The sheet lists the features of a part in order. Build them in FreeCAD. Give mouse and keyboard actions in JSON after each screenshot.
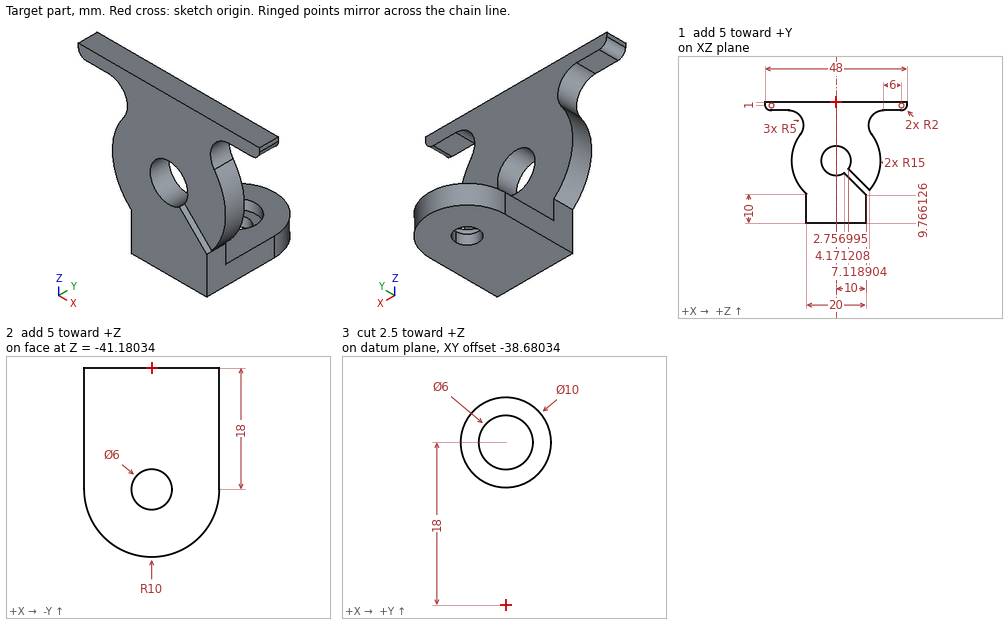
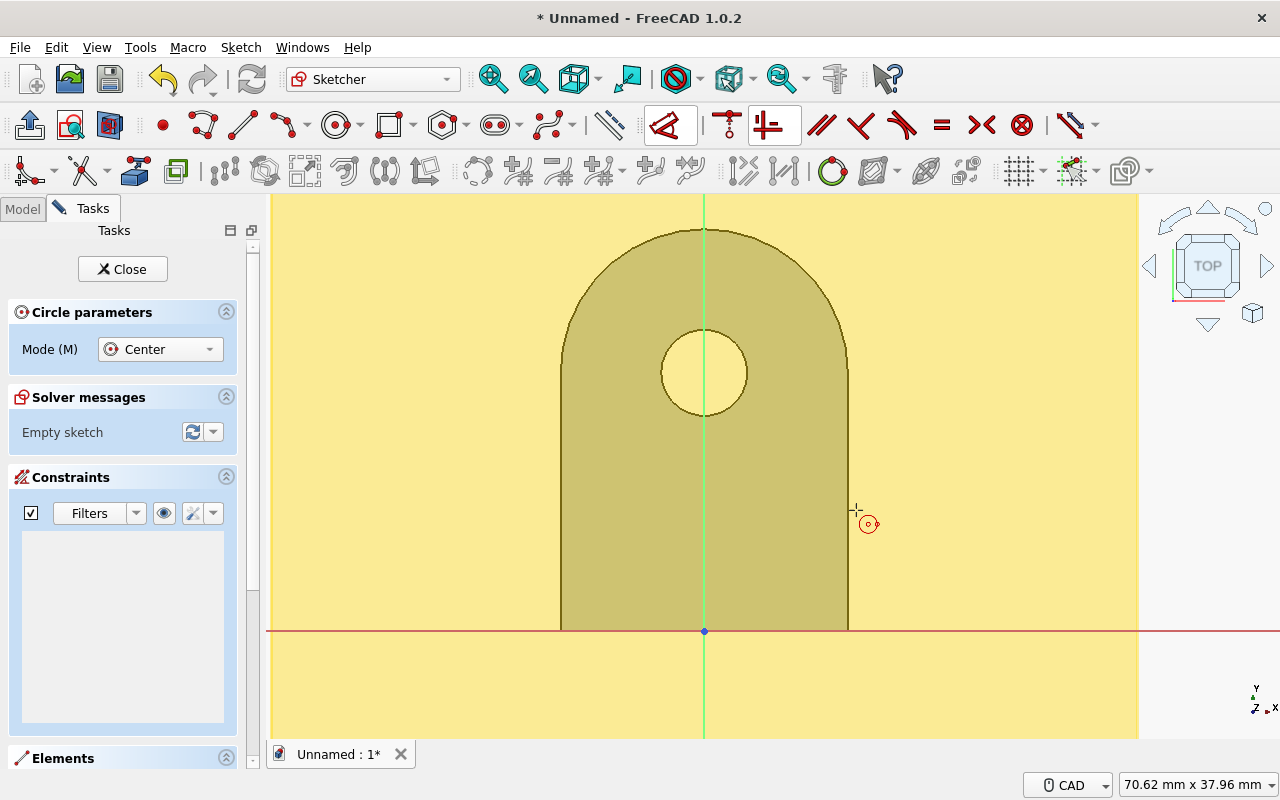
{"action": "left_click", "coordinate": [704, 373]}
{"action": "left_click", "coordinate": [755, 322]}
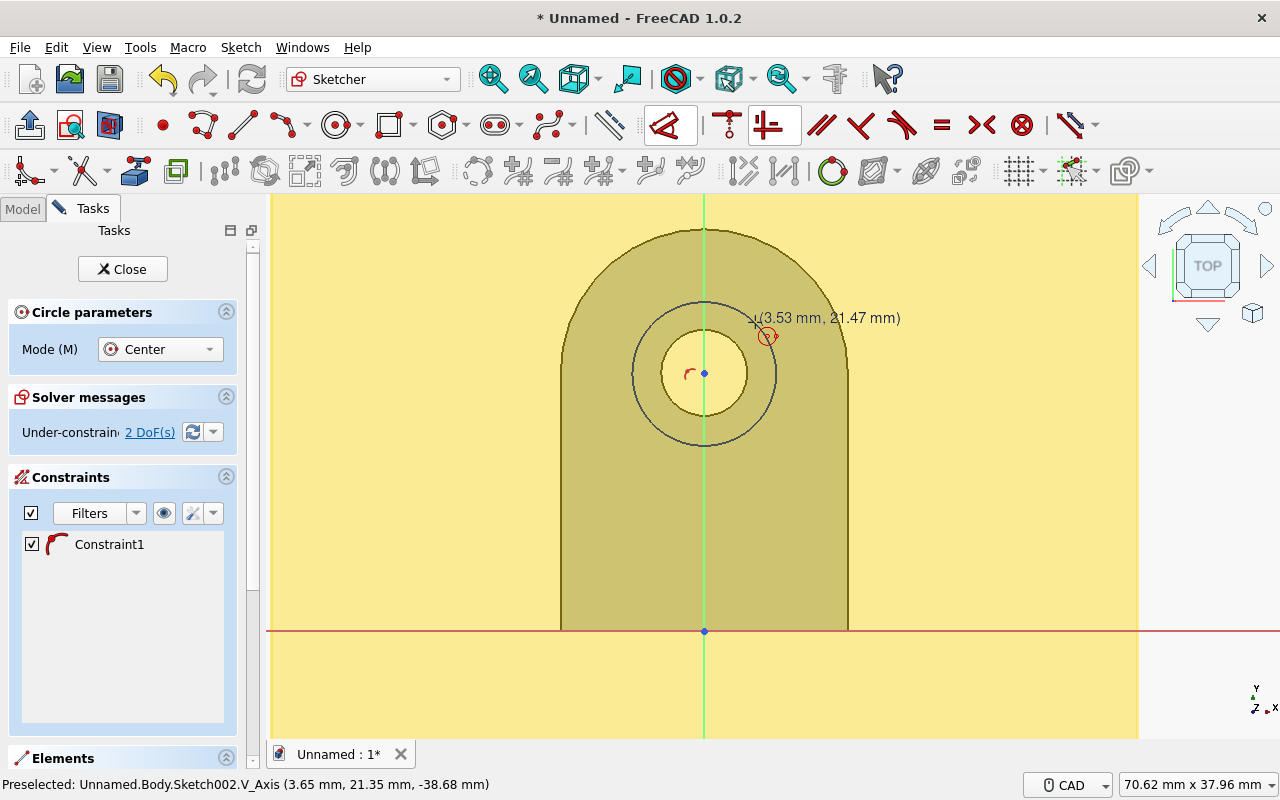
{"action": "left_click", "coordinate": [704, 374]}
{"action": "left_click", "coordinate": [735, 342]}
{"action": "key", "text": "Escape"}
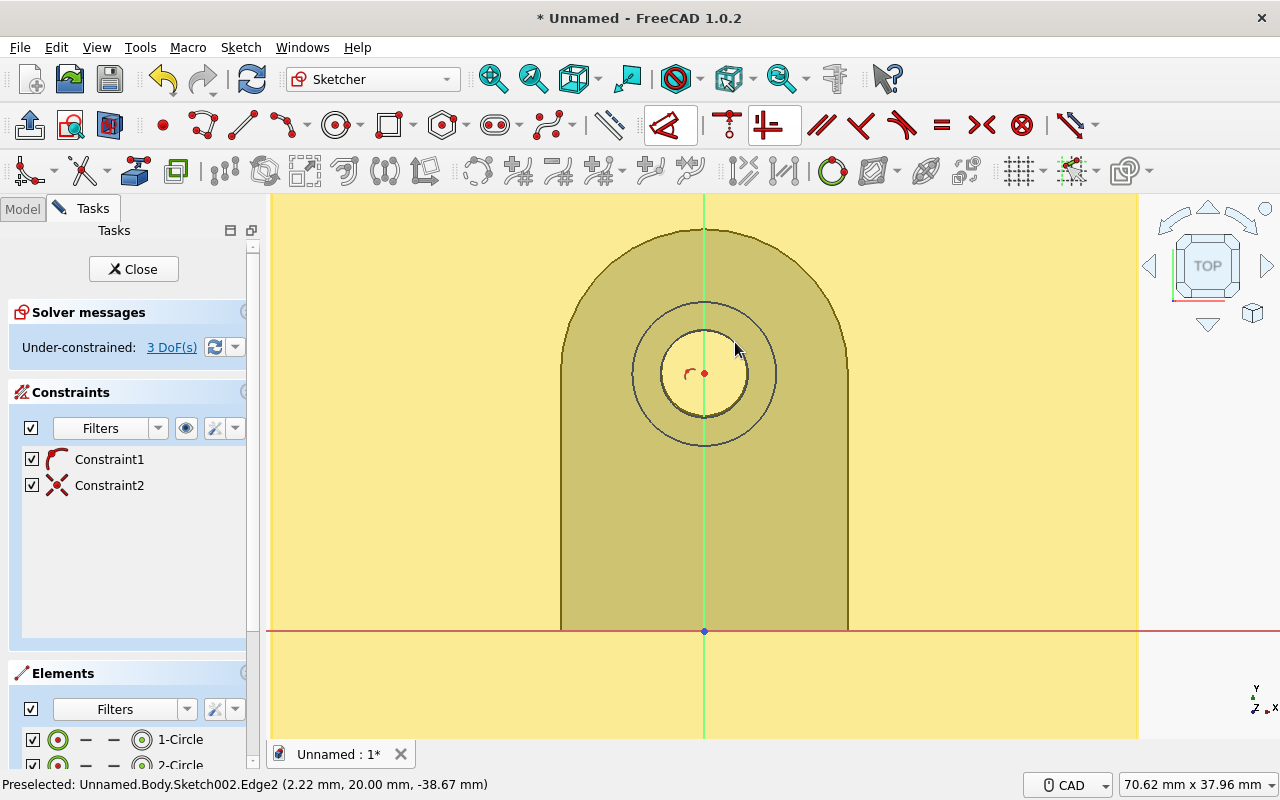
{"action": "left_click", "coordinate": [755, 323]}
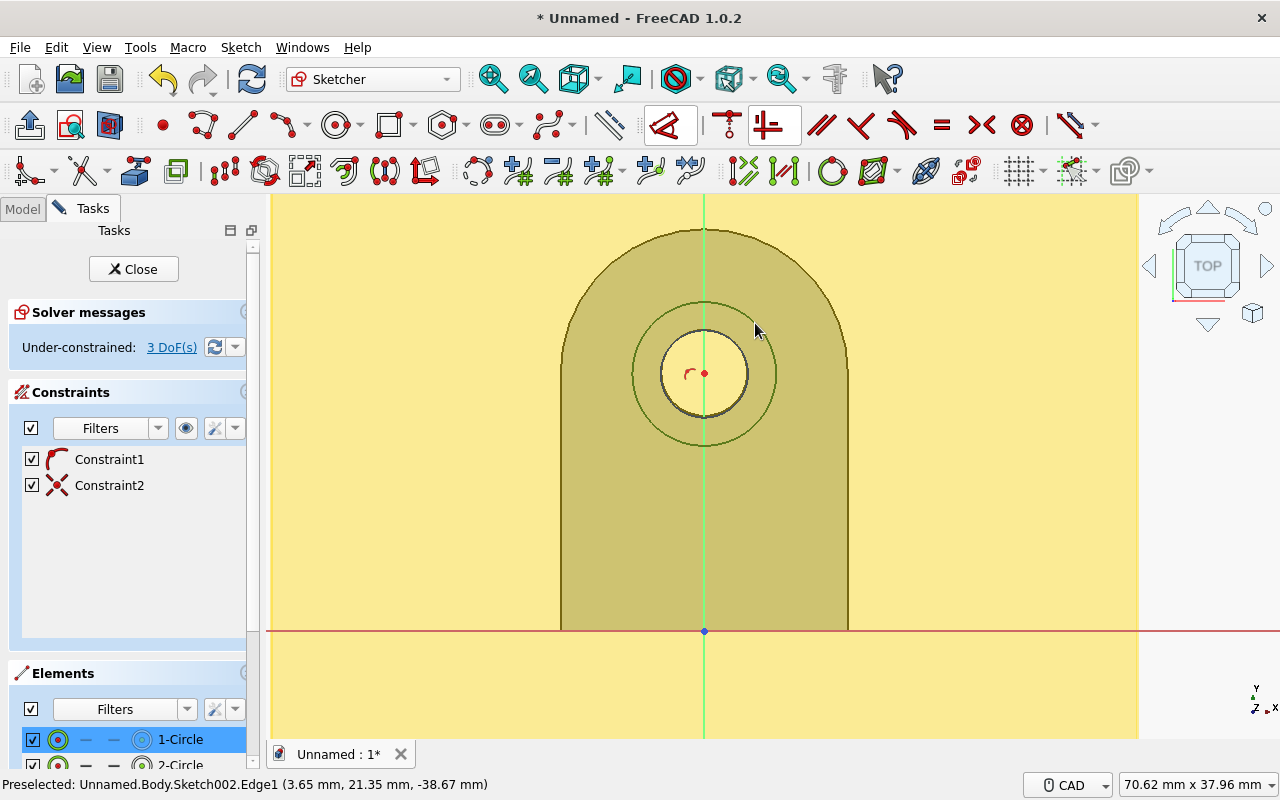
{"action": "left_click", "coordinate": [692, 126]}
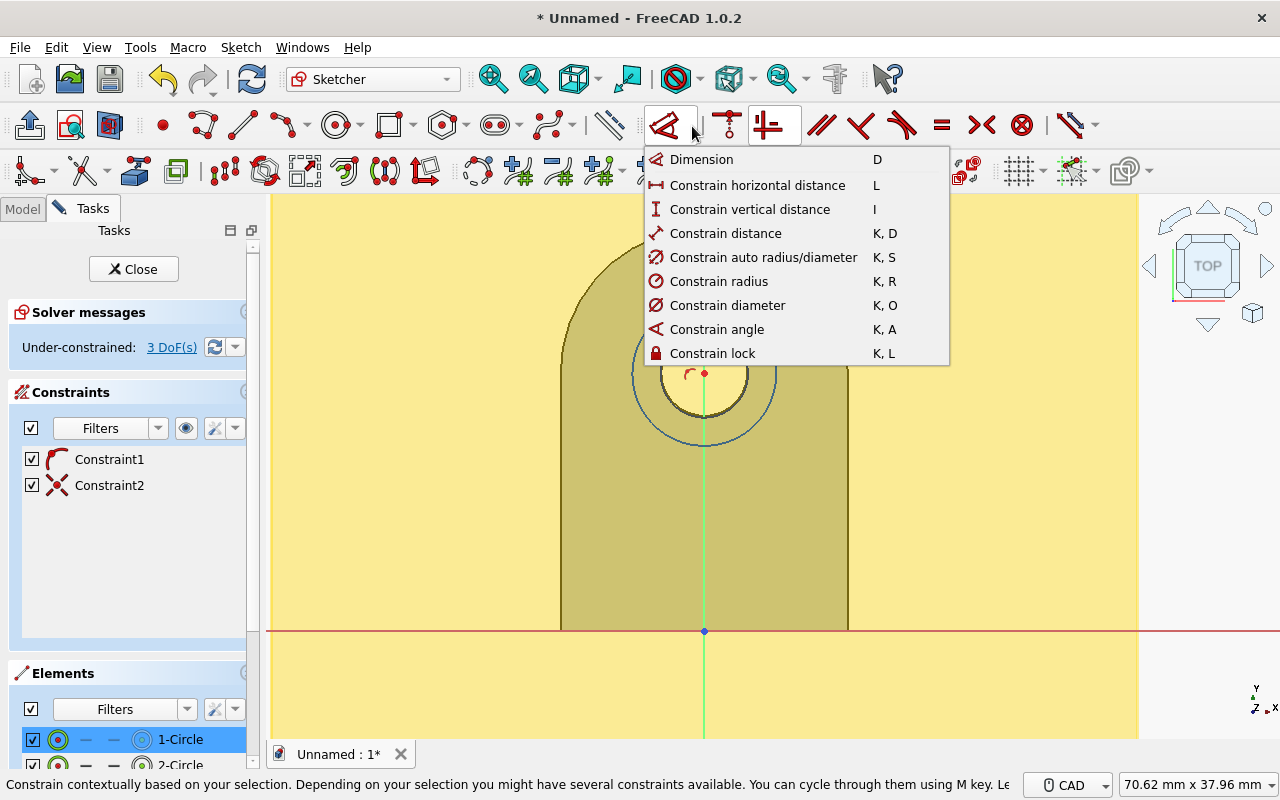
{"action": "left_click", "coordinate": [797, 305]}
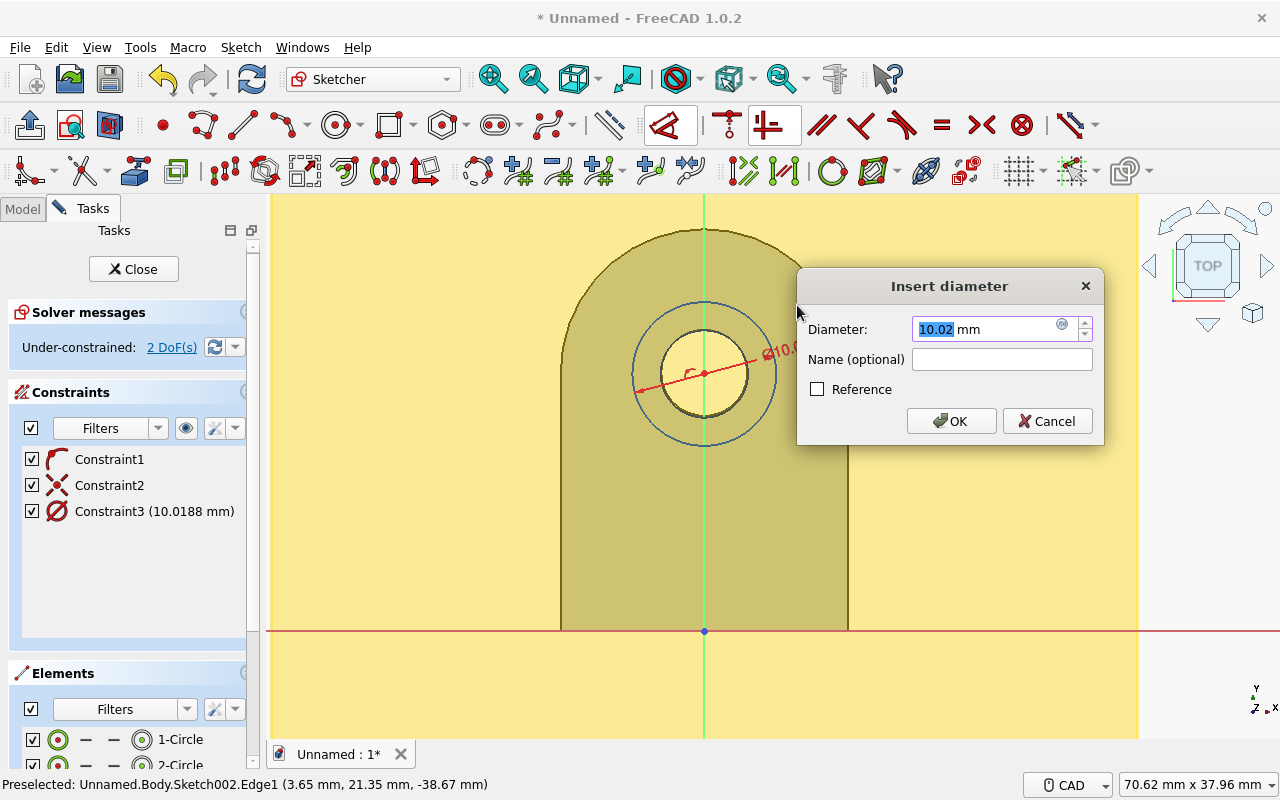
{"action": "type", "text": "10"}
{"action": "key", "text": "Return"}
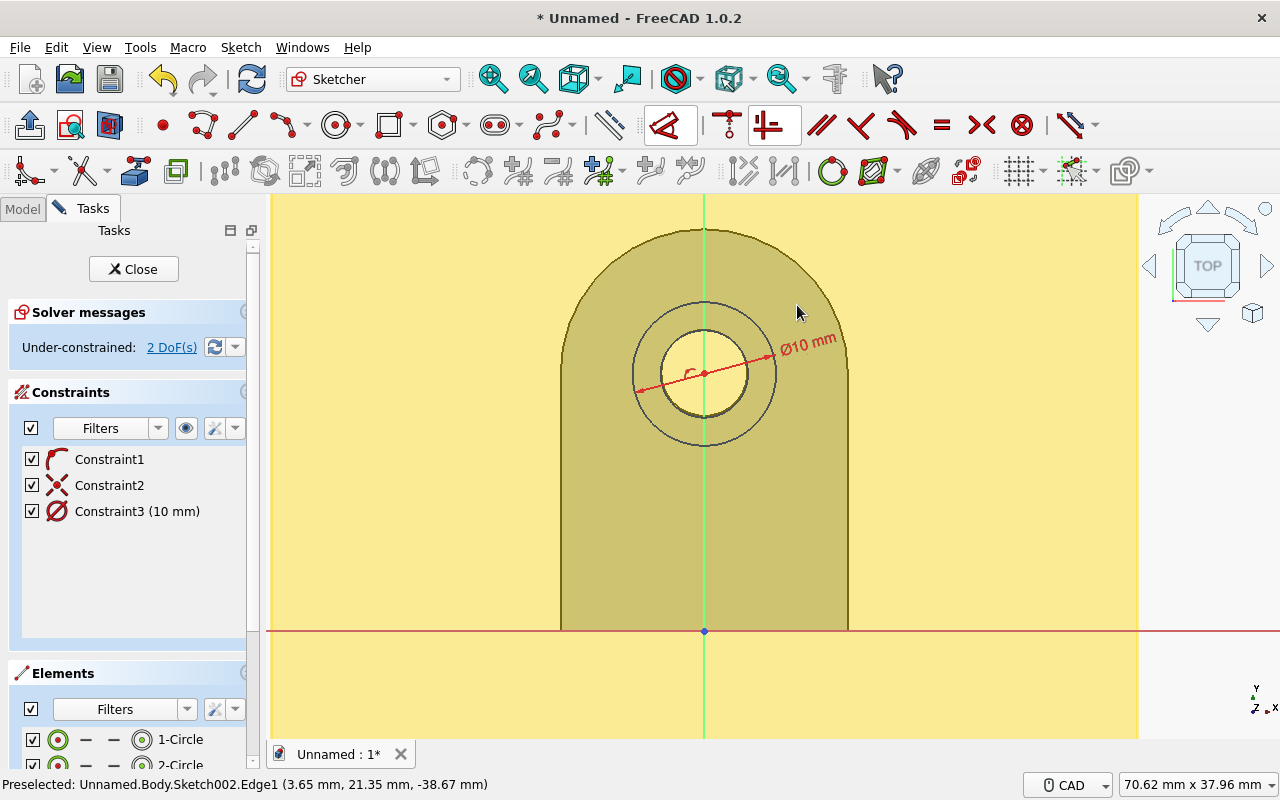
{"action": "left_click", "coordinate": [735, 343]}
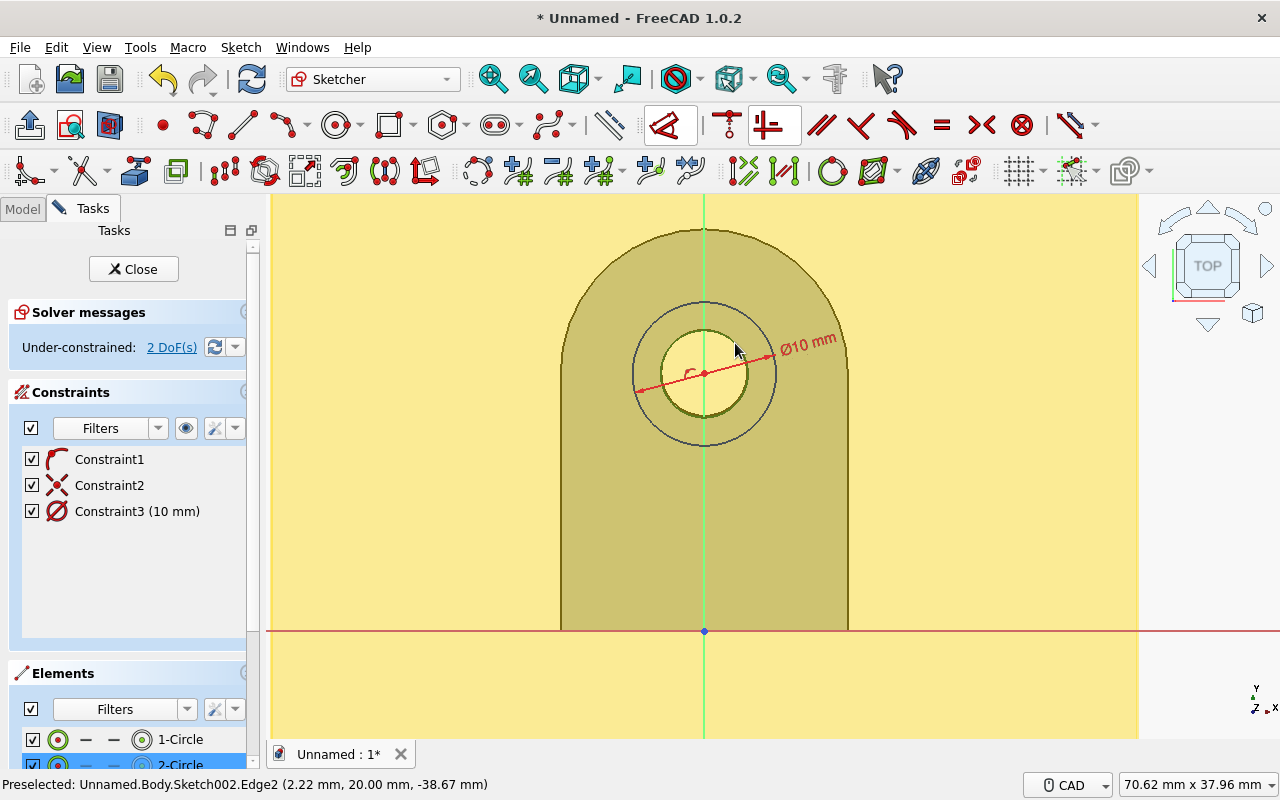
{"action": "key", "text": "k o"}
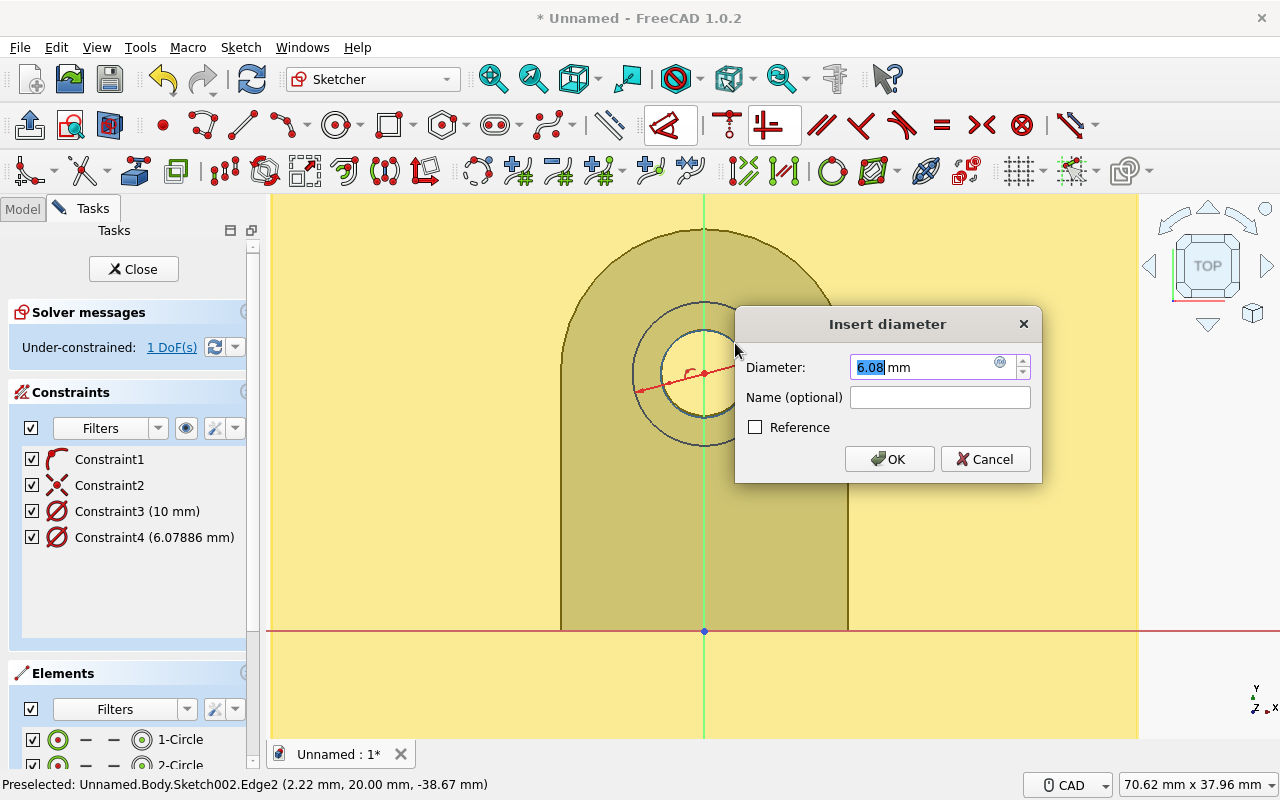
{"action": "type", "text": "6"}
{"action": "key", "text": "Return"}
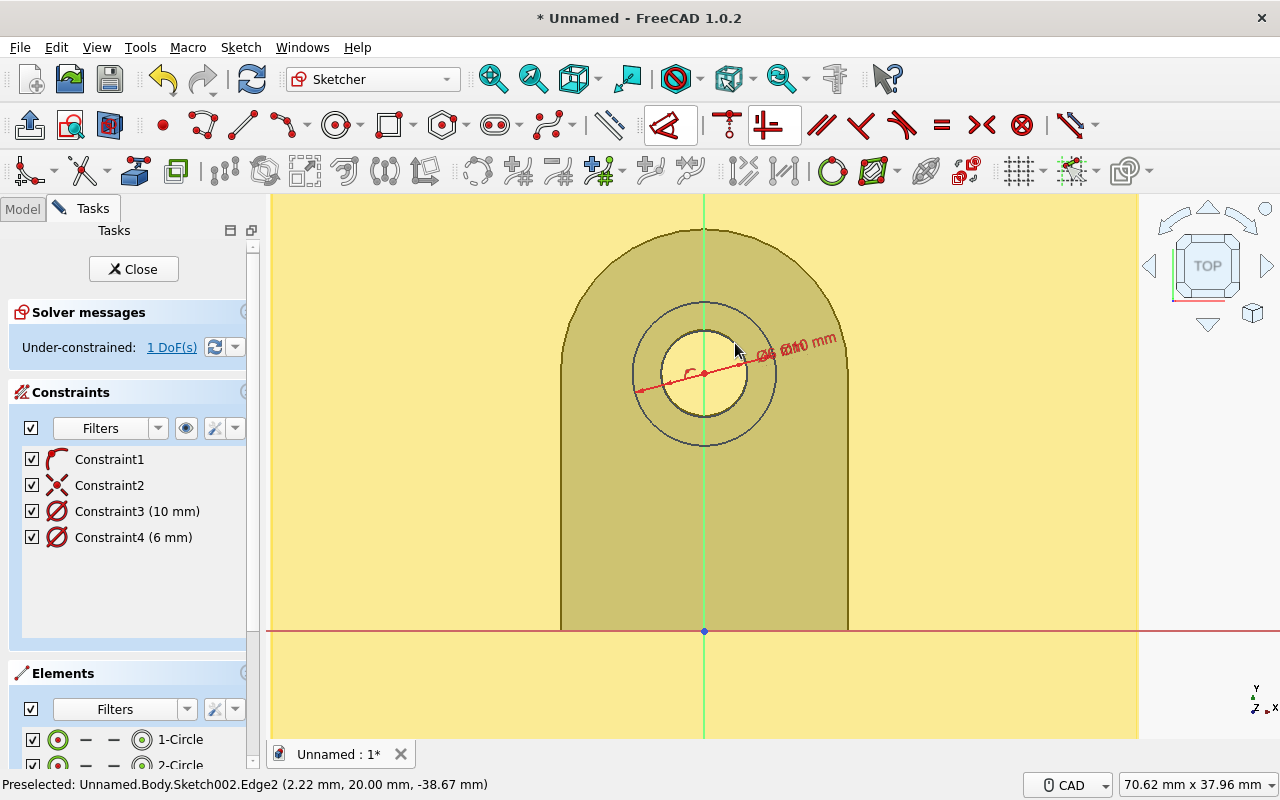
{"action": "left_click", "coordinate": [704, 374]}